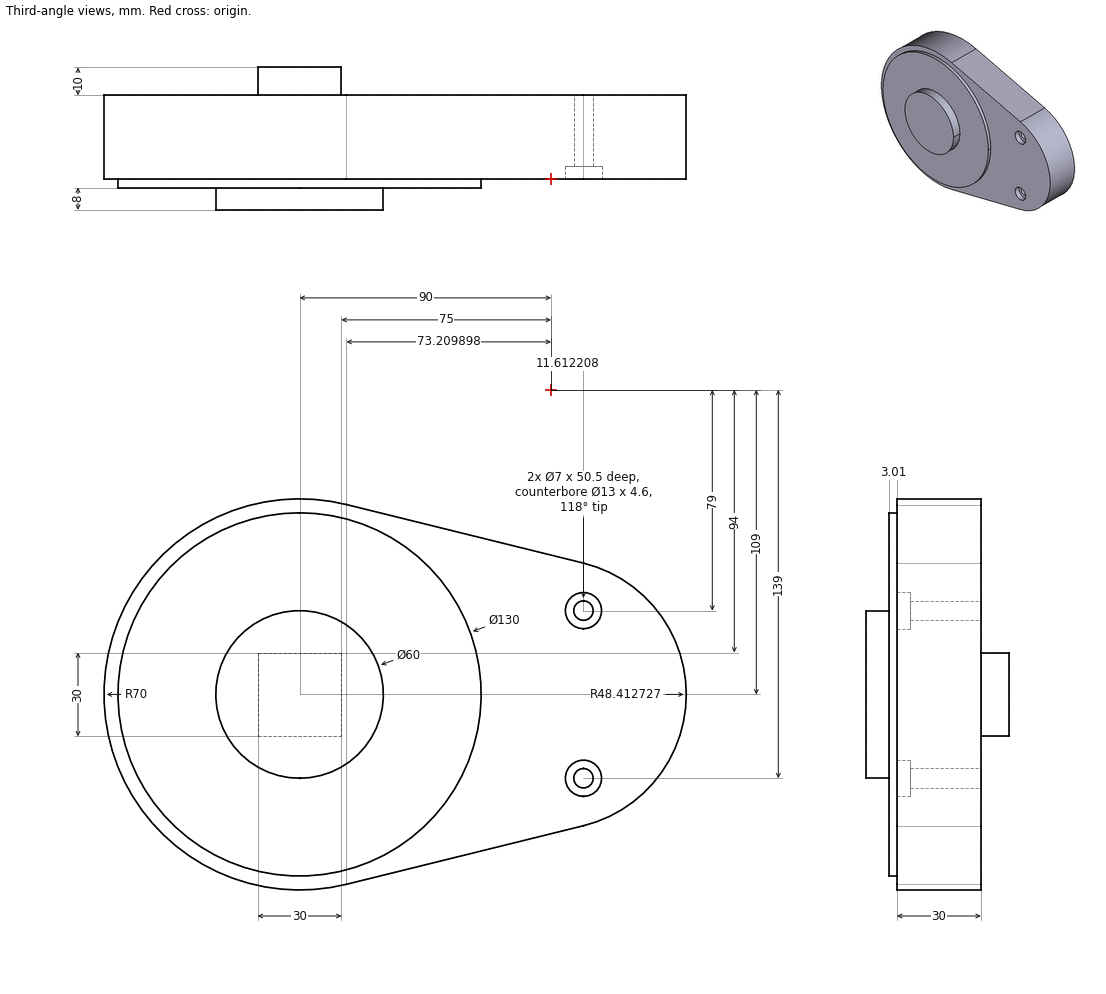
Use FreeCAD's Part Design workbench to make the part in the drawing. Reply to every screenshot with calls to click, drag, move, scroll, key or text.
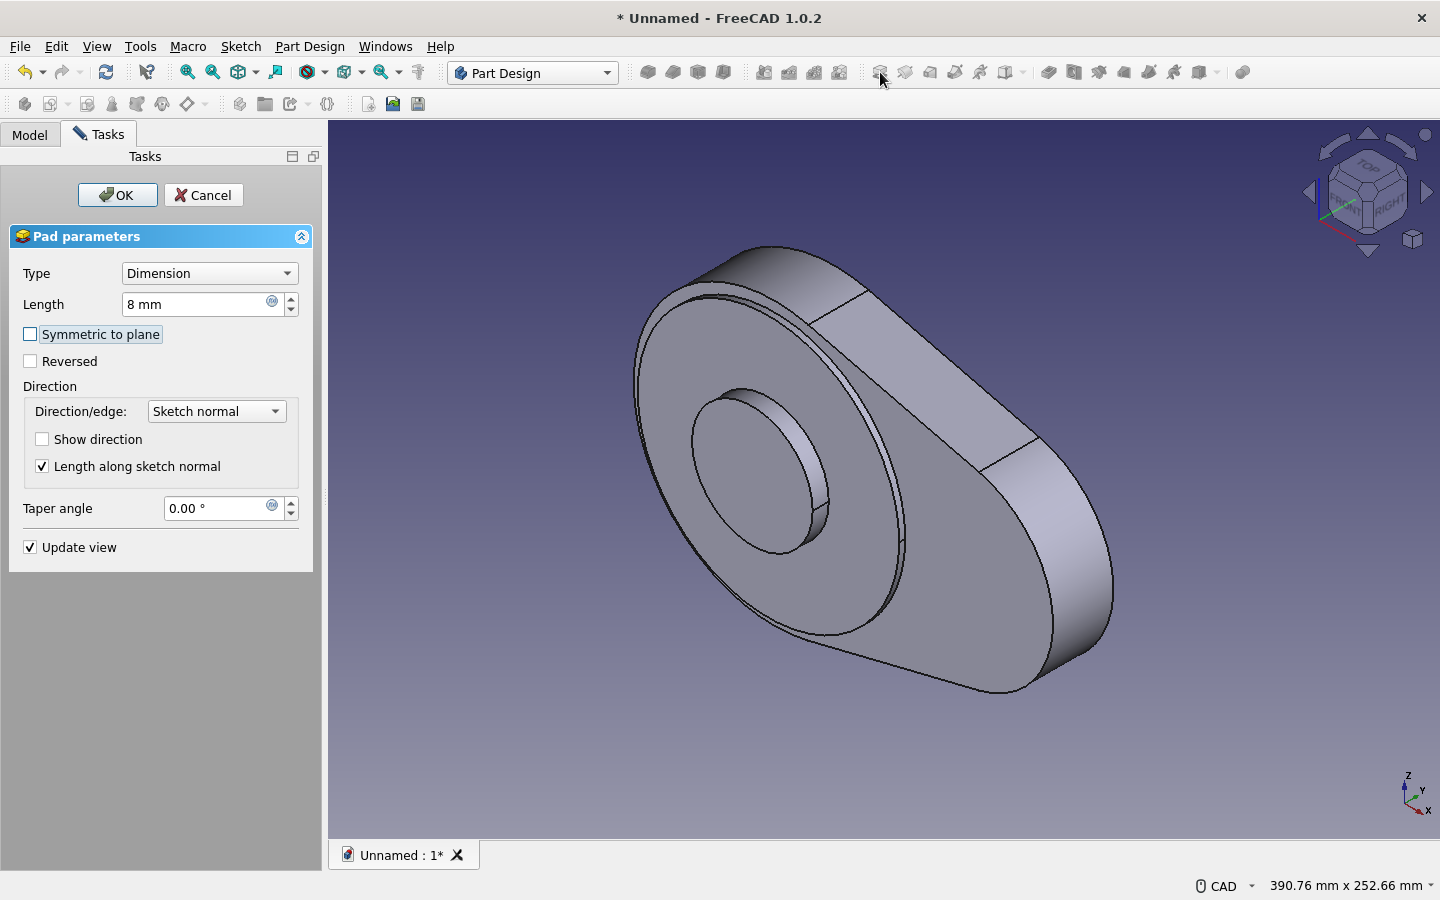
click(118, 195)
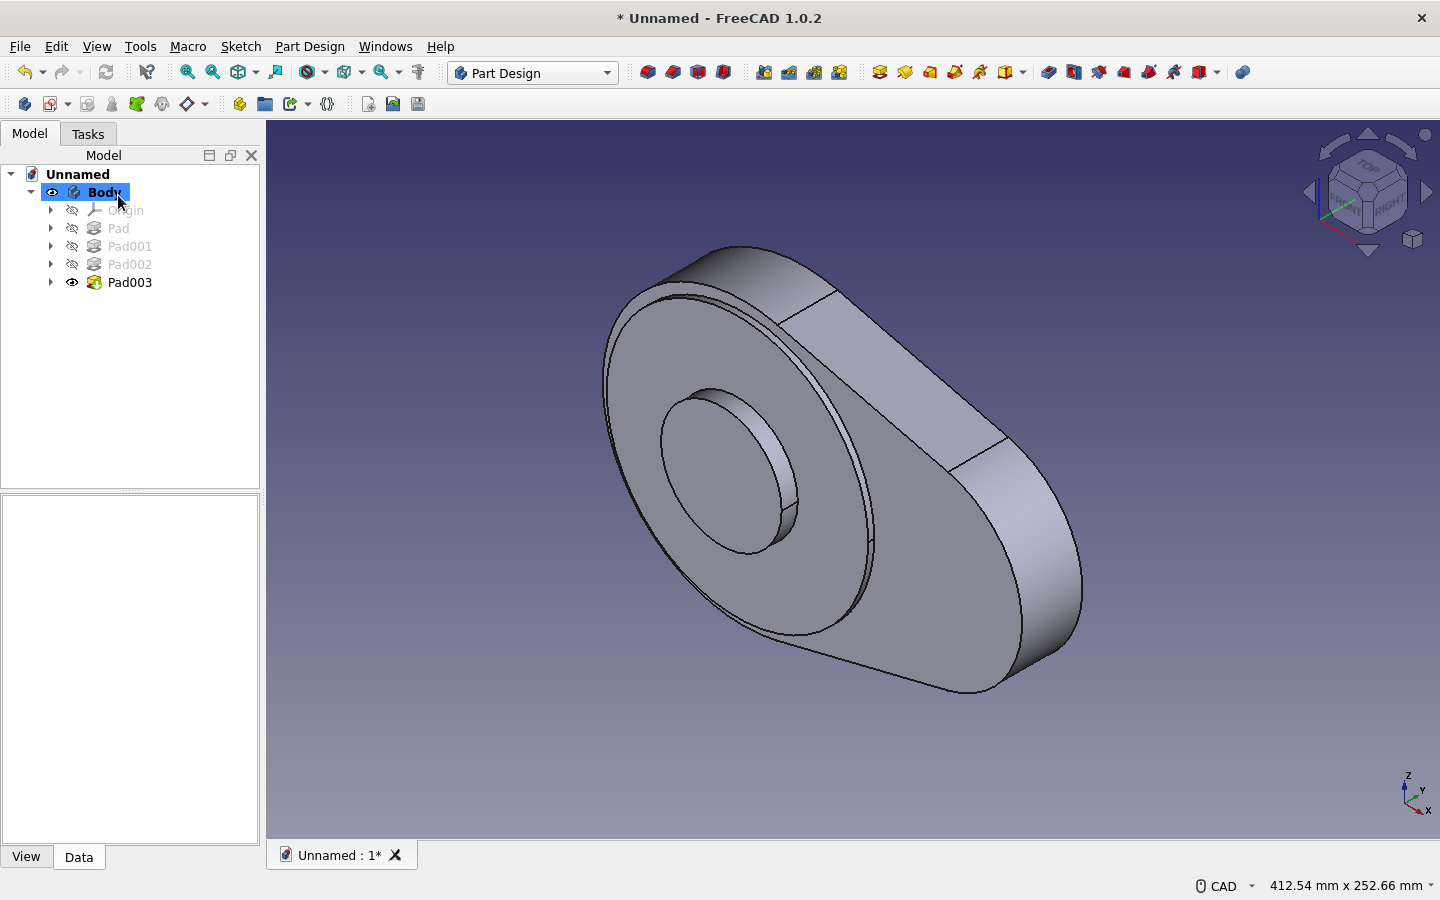
click(50, 104)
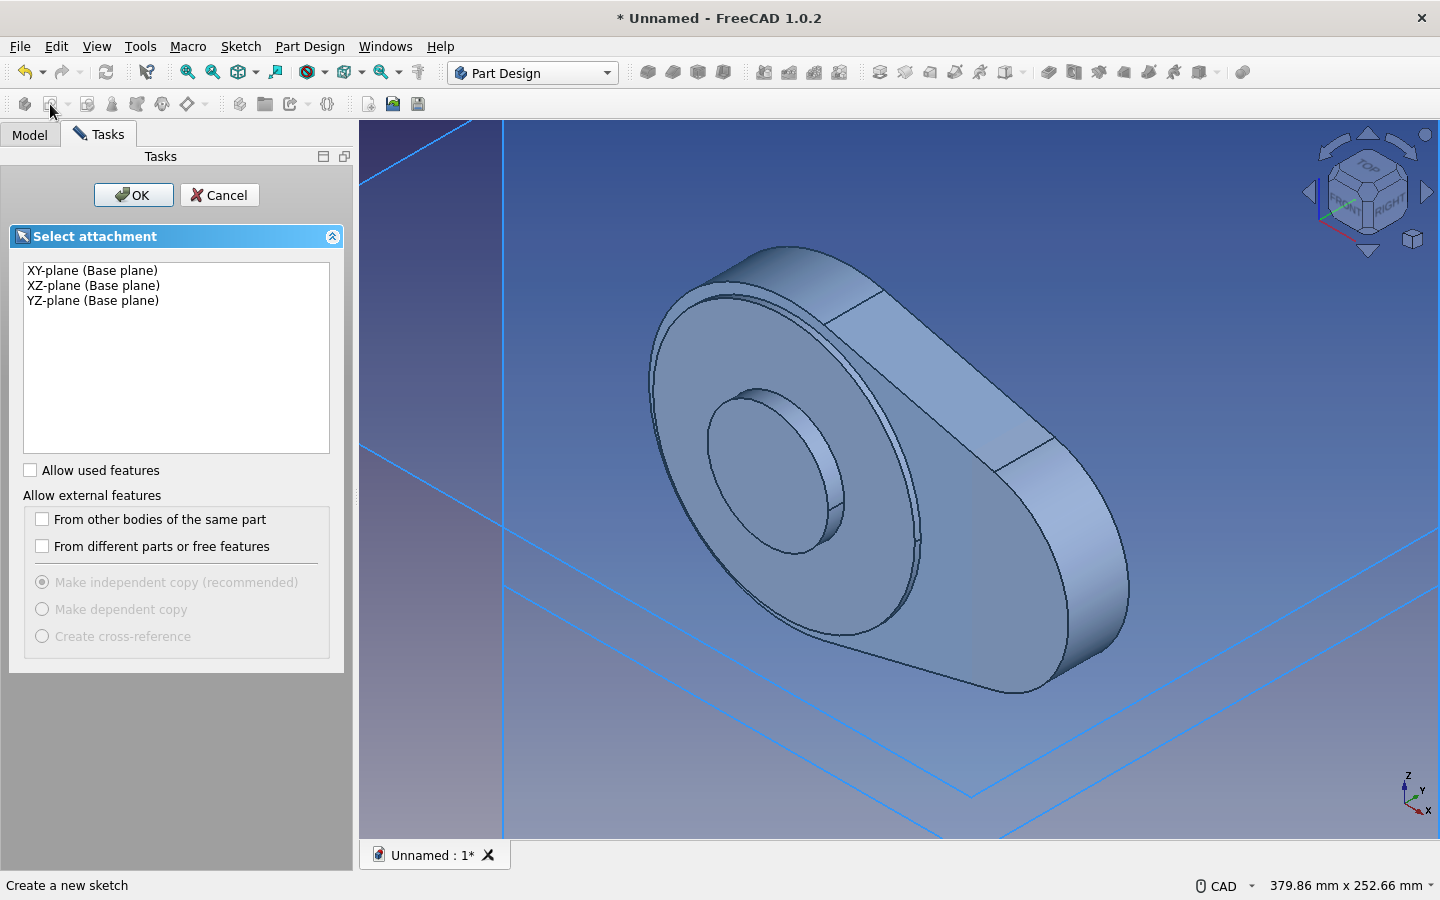
click(84, 286)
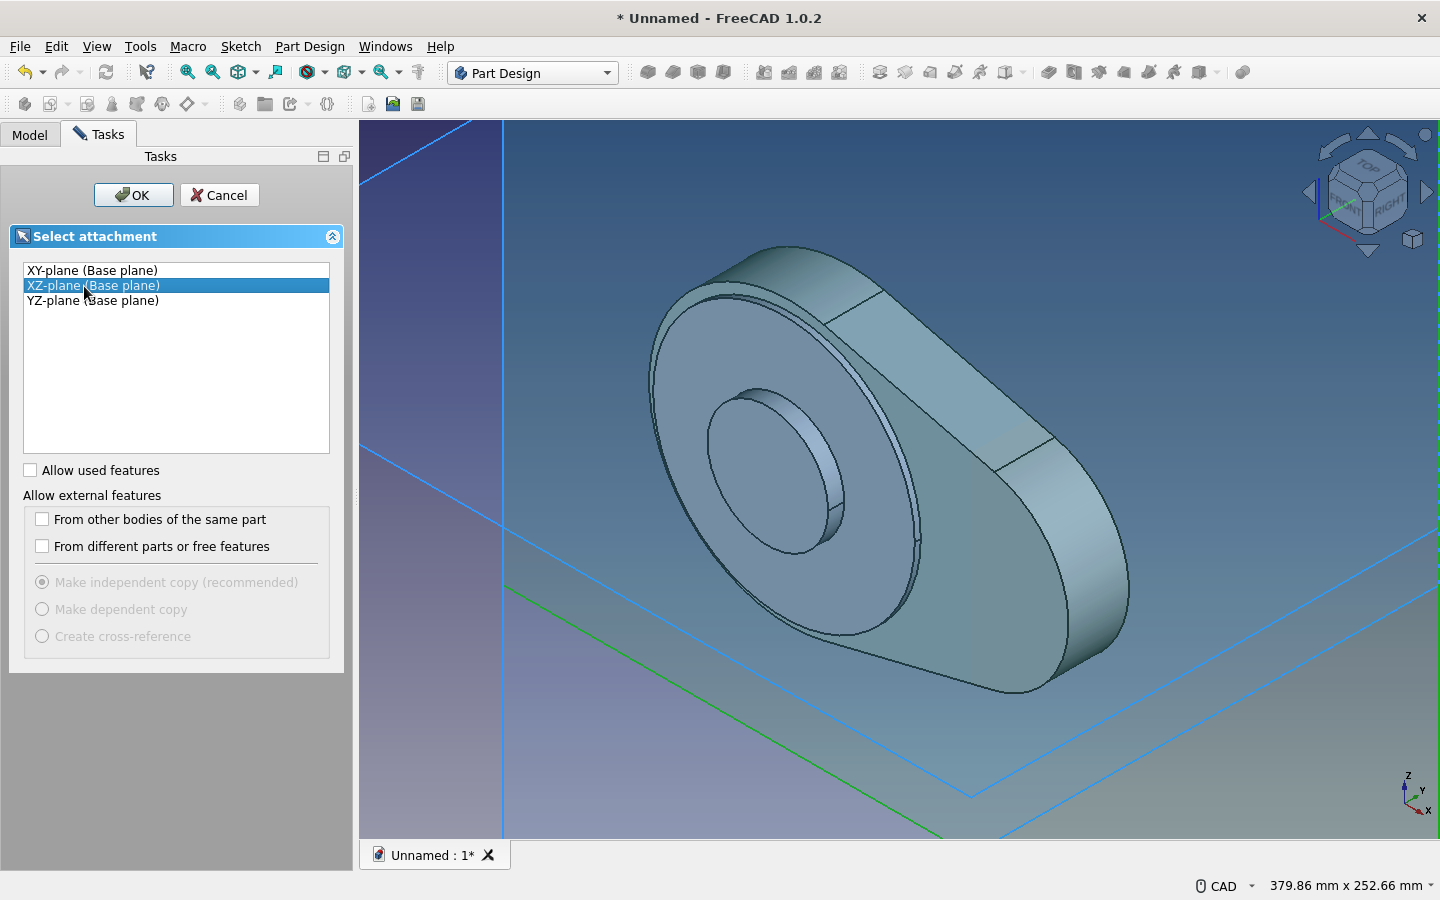
click(134, 195)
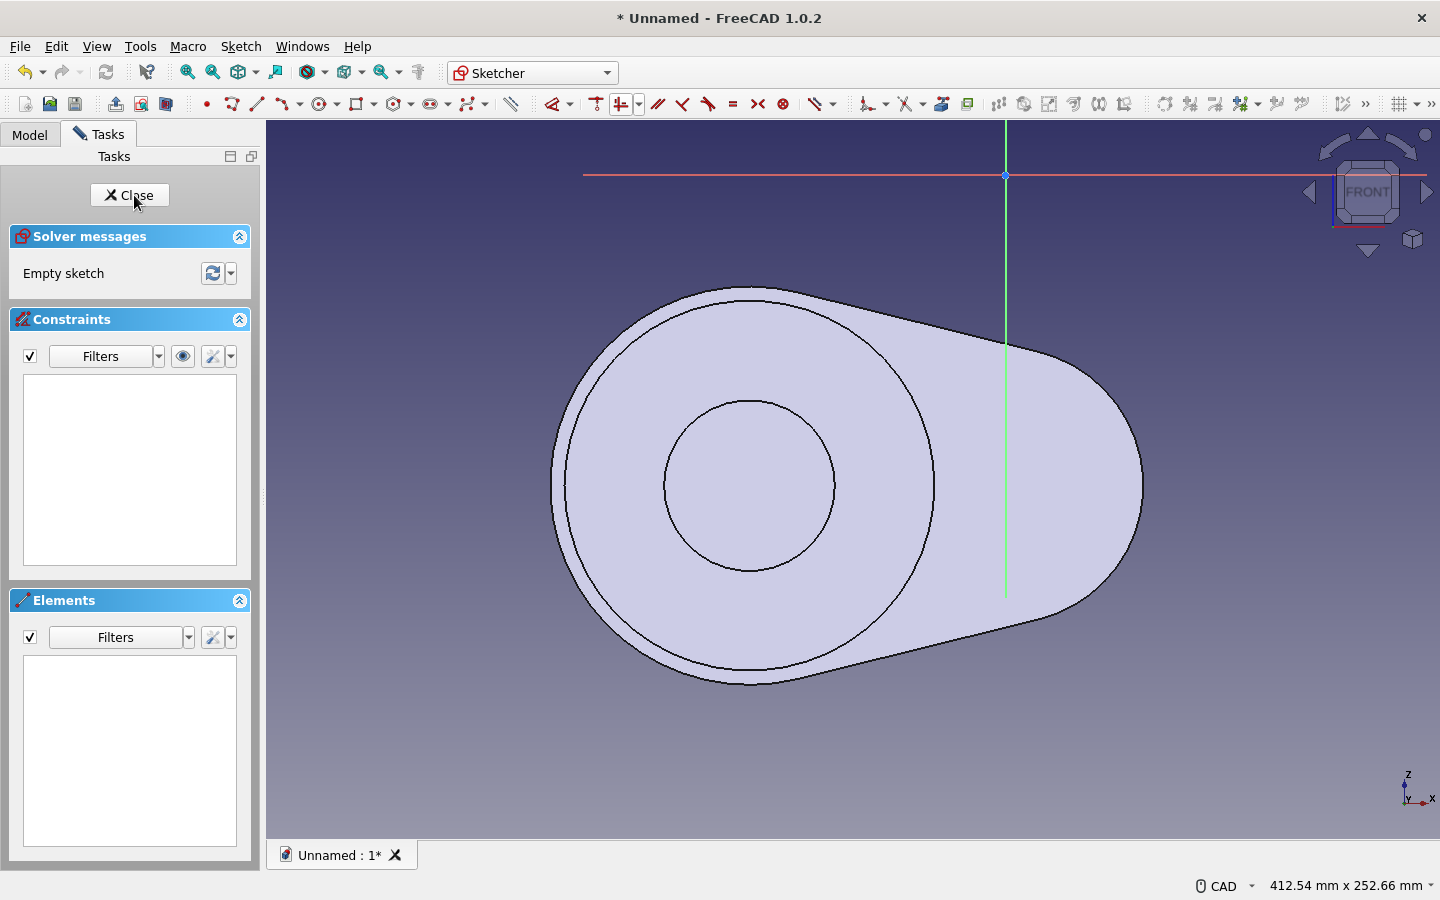
click(166, 104)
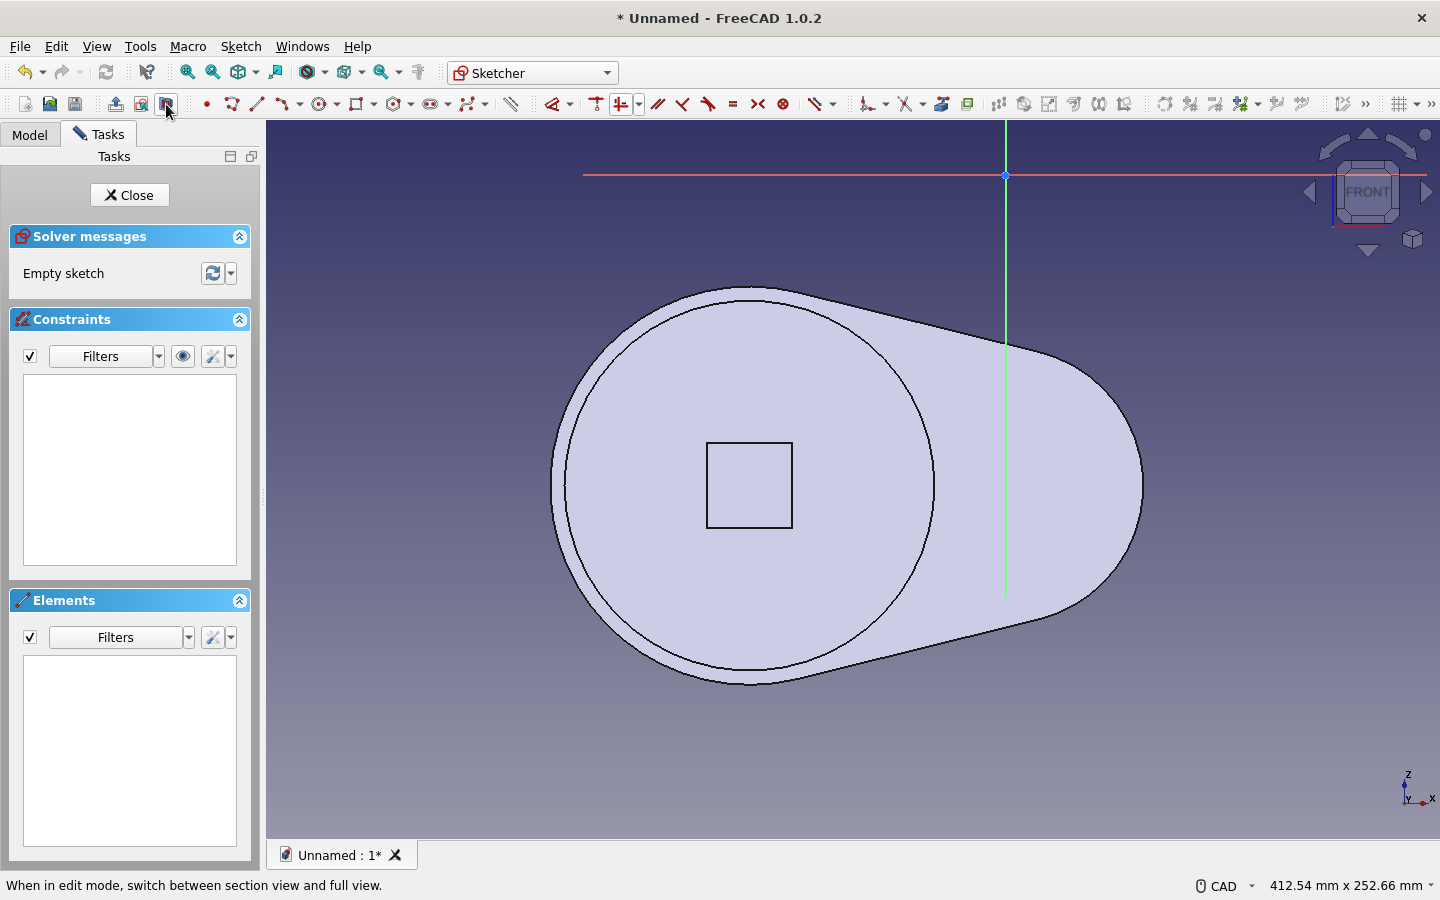
key(g)
key(c)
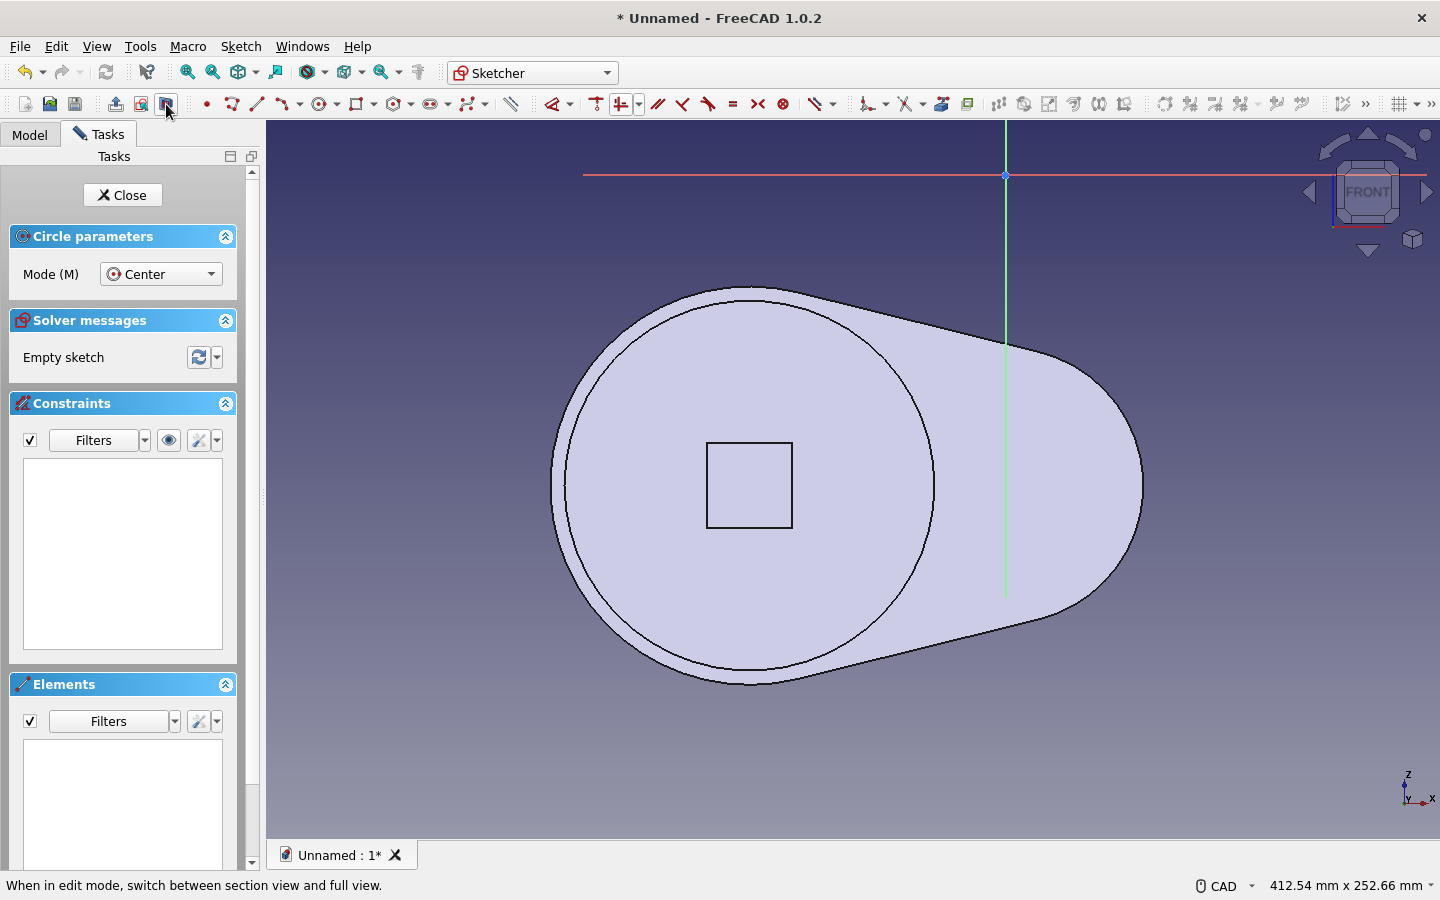
scroll(1039, 400, up, 5)